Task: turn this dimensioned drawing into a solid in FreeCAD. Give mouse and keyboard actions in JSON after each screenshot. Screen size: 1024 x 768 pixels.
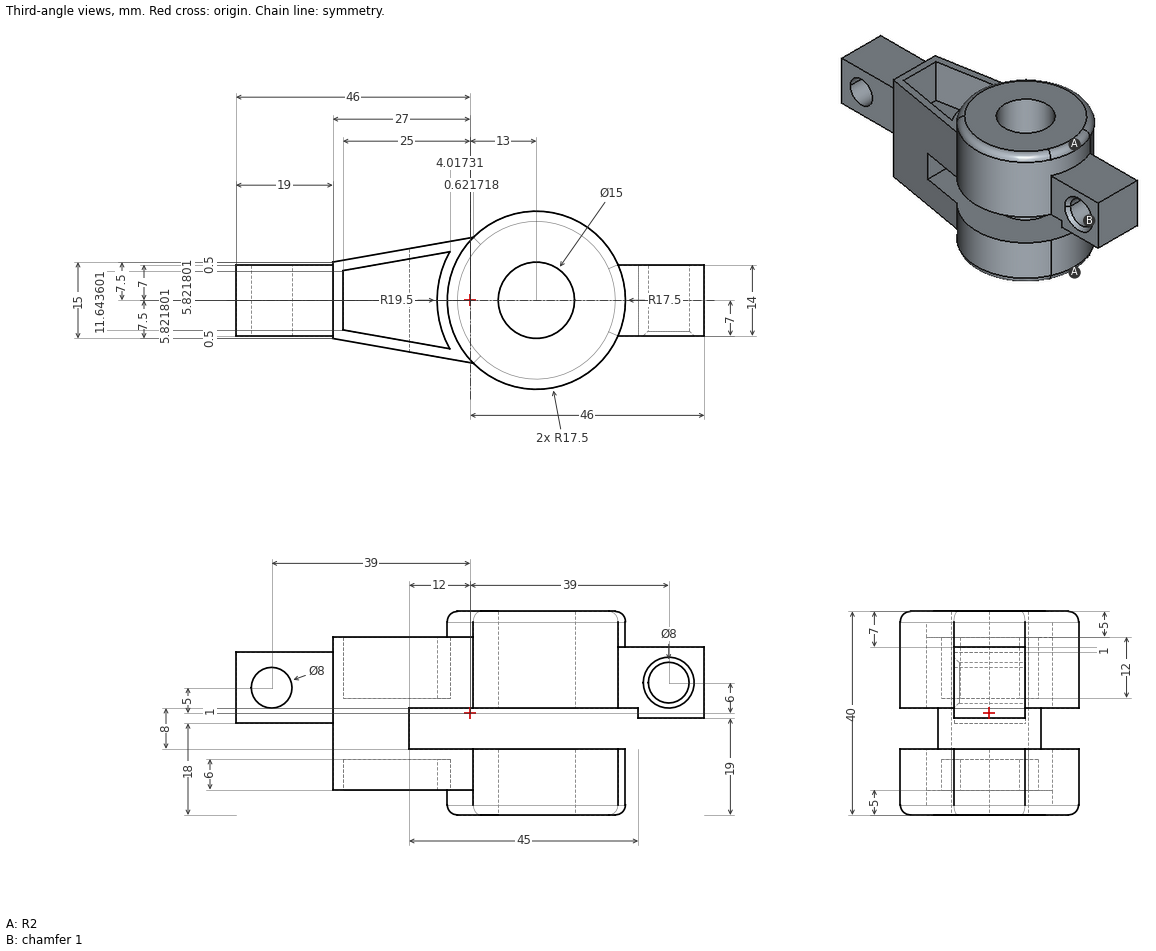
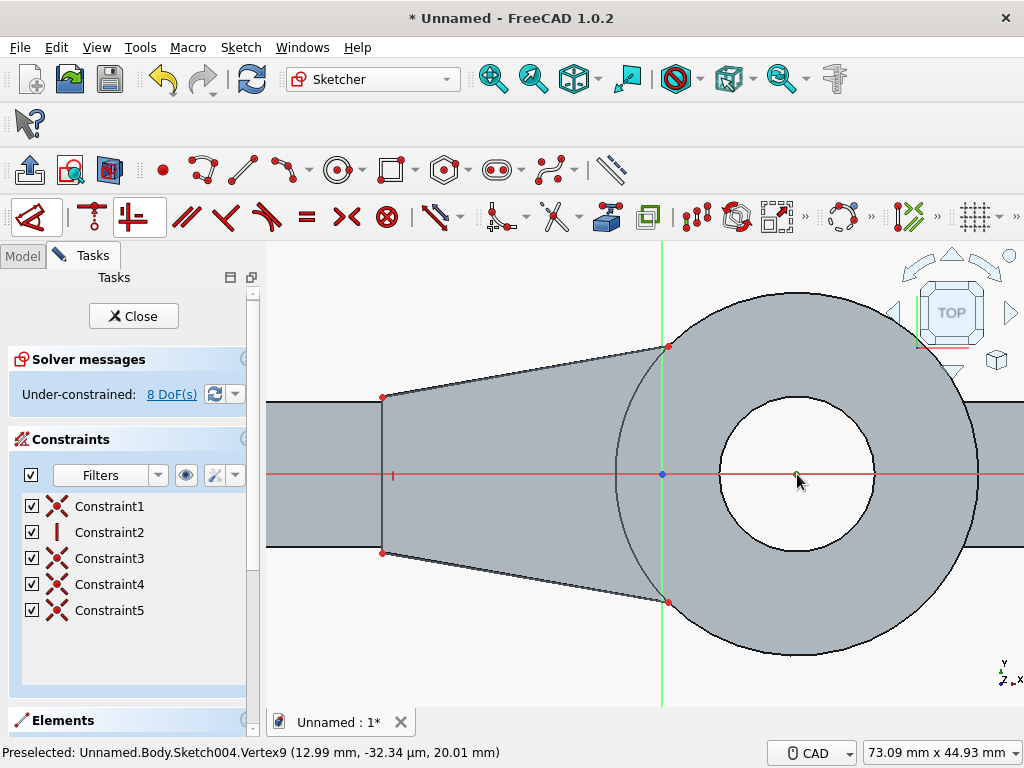
{"action": "left_click", "coordinate": [334, 474]}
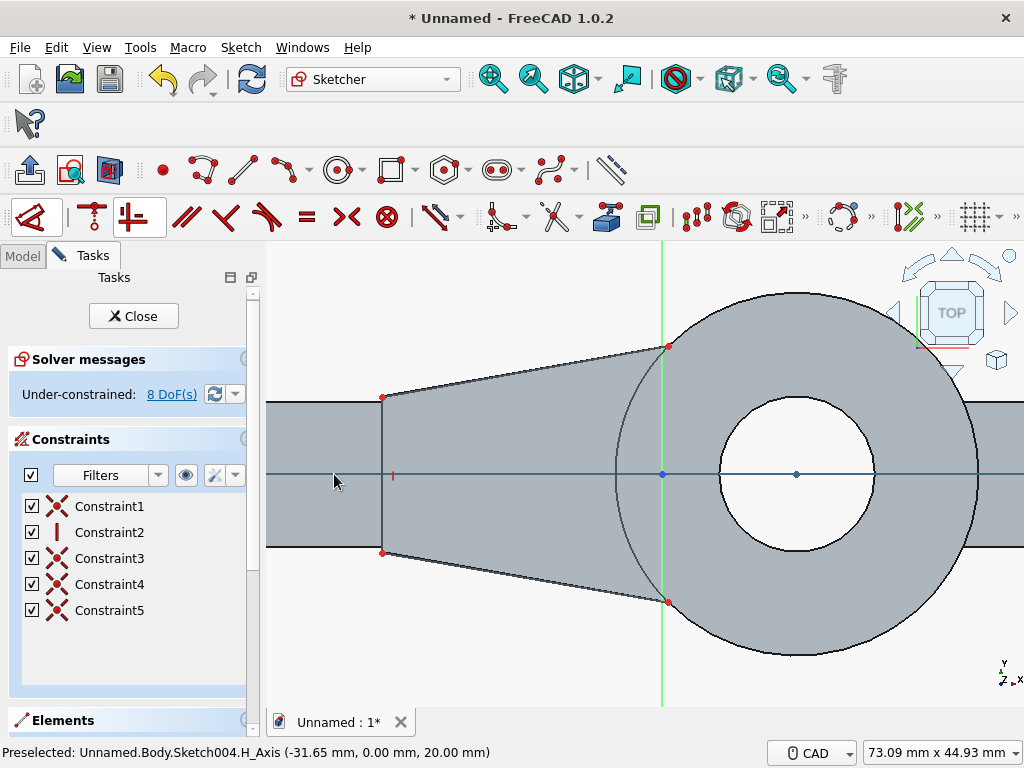
{"action": "left_click", "coordinate": [92, 218]}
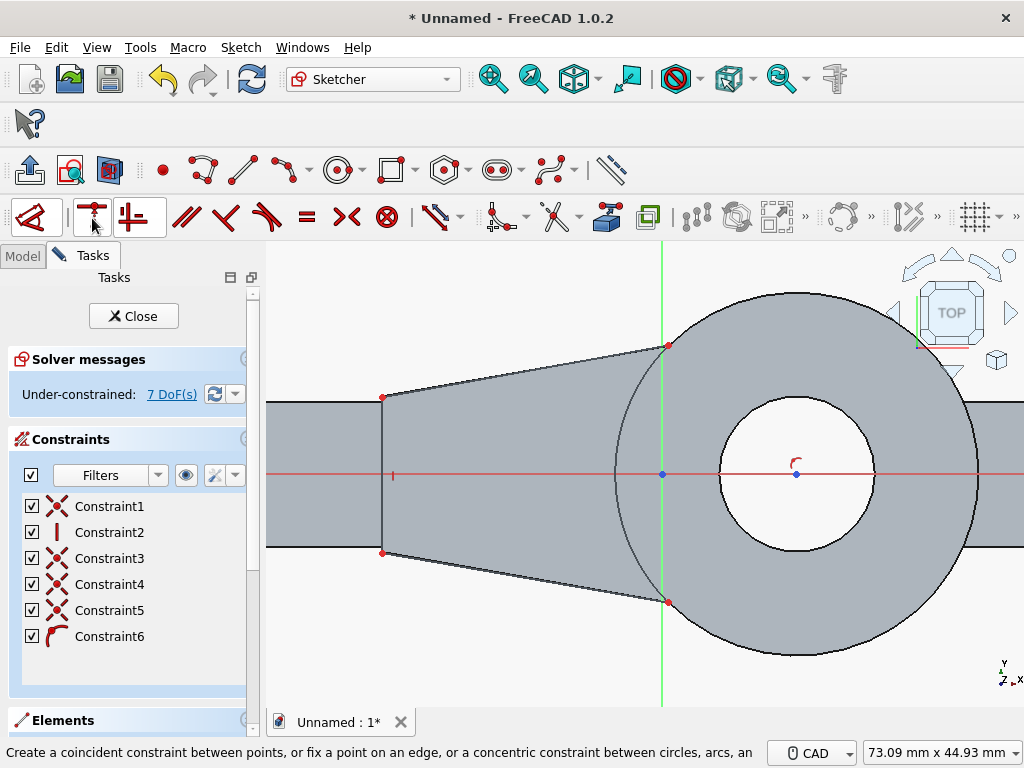
{"action": "left_click", "coordinate": [624, 418]}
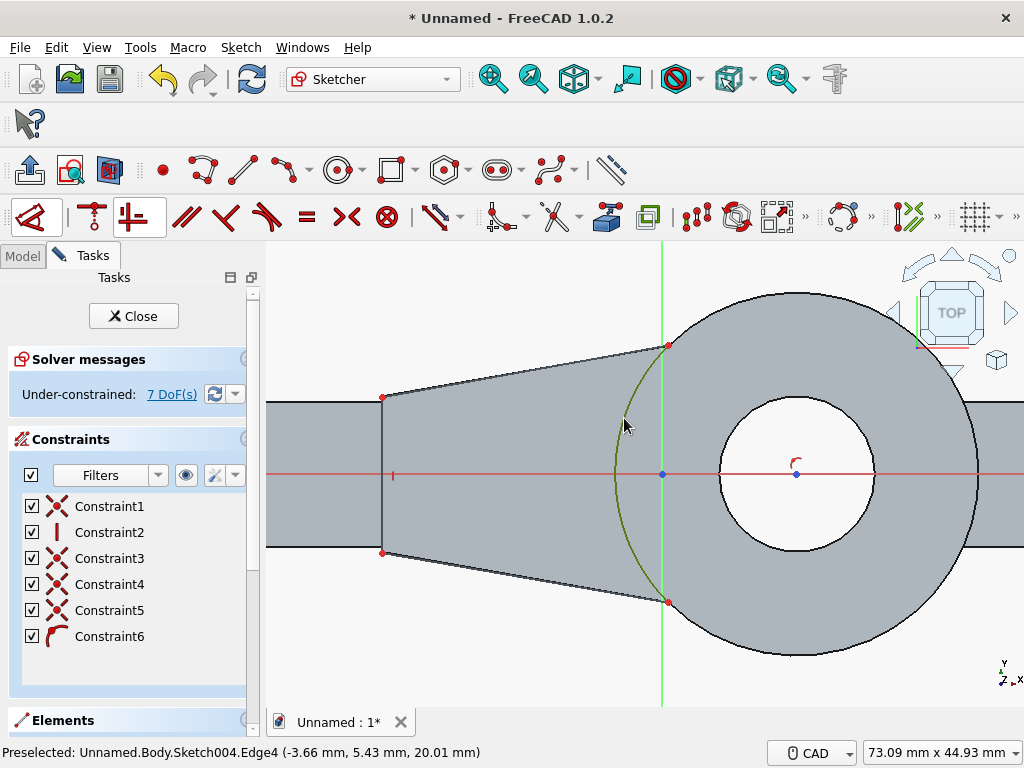
{"action": "key", "text": "k r"}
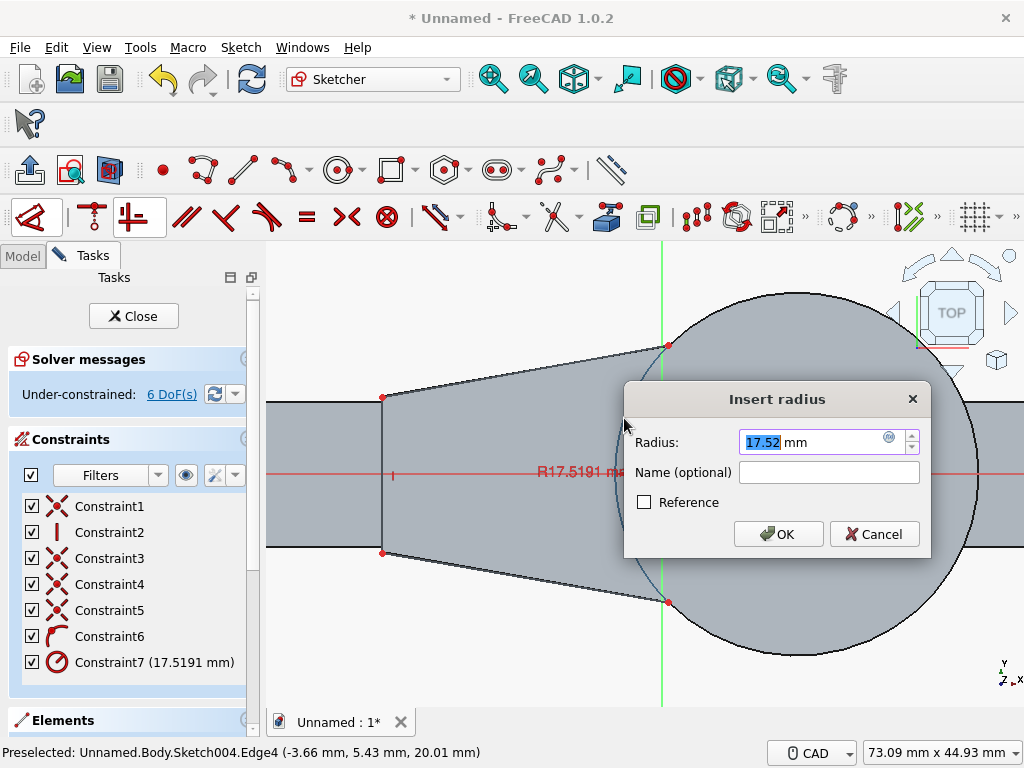
{"action": "type", "text": "17.5"}
{"action": "key", "text": "Return"}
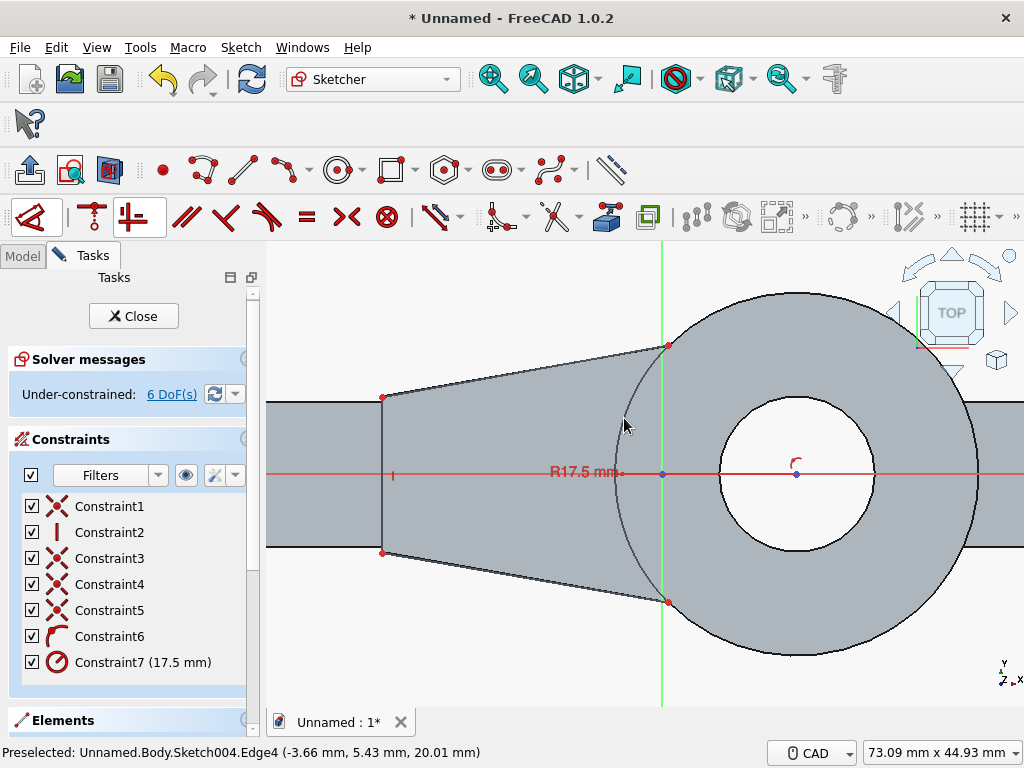
{"action": "left_click", "coordinate": [382, 444]}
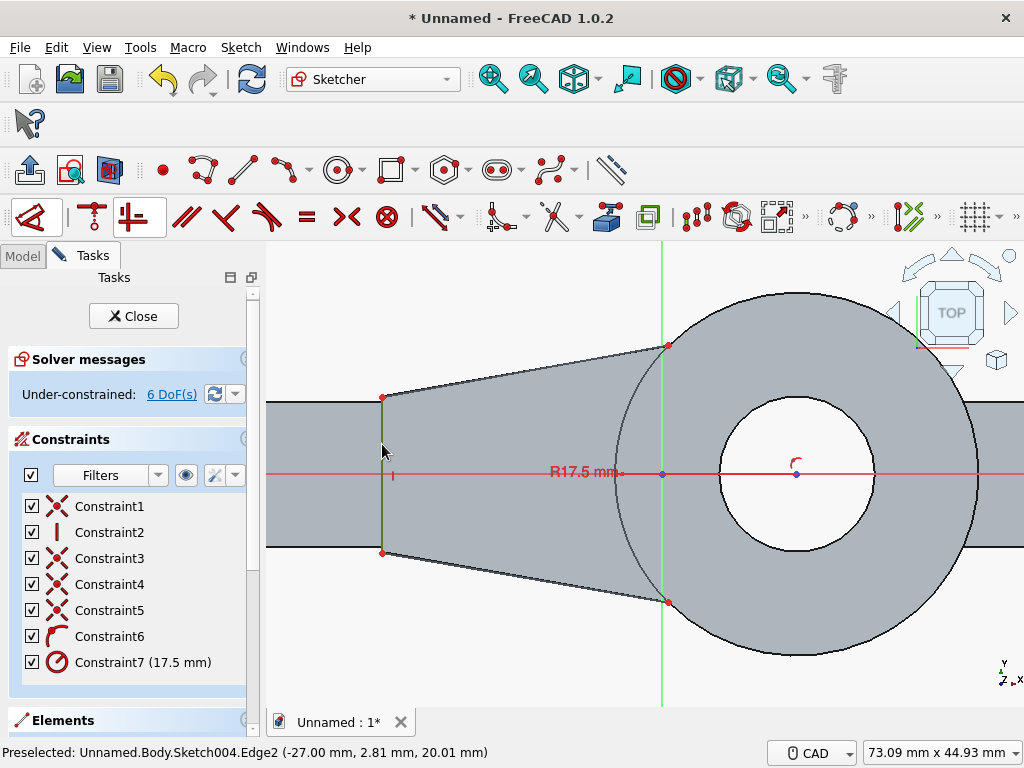
{"action": "left_click", "coordinate": [56, 218]}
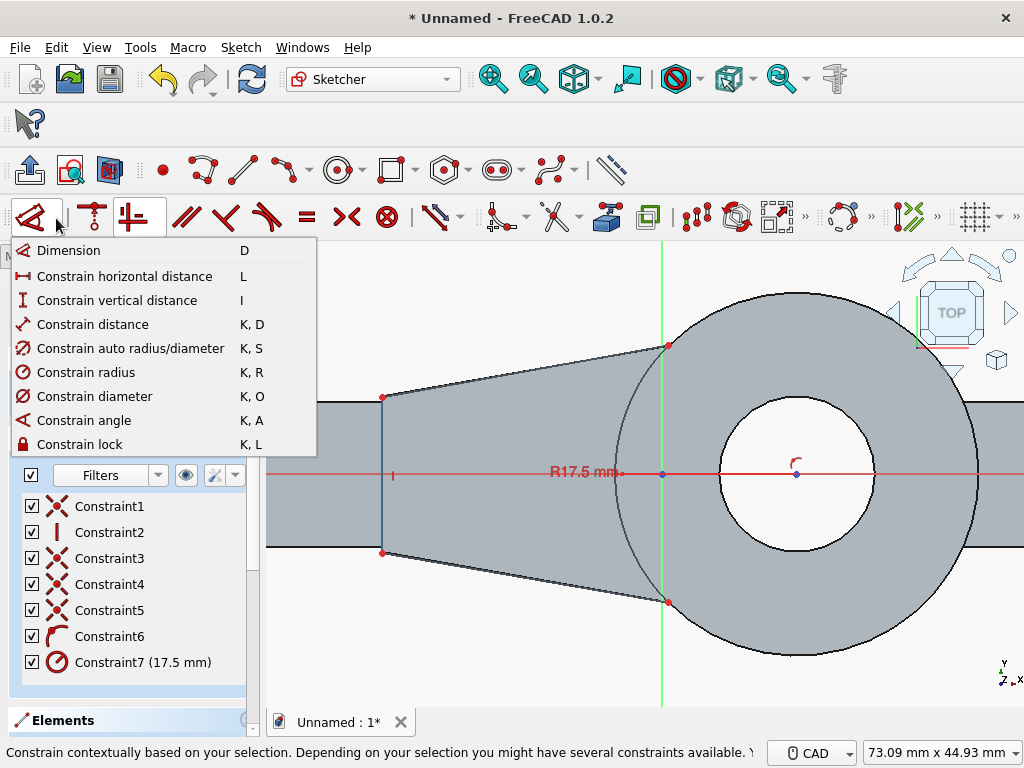
{"action": "left_click", "coordinate": [164, 300]}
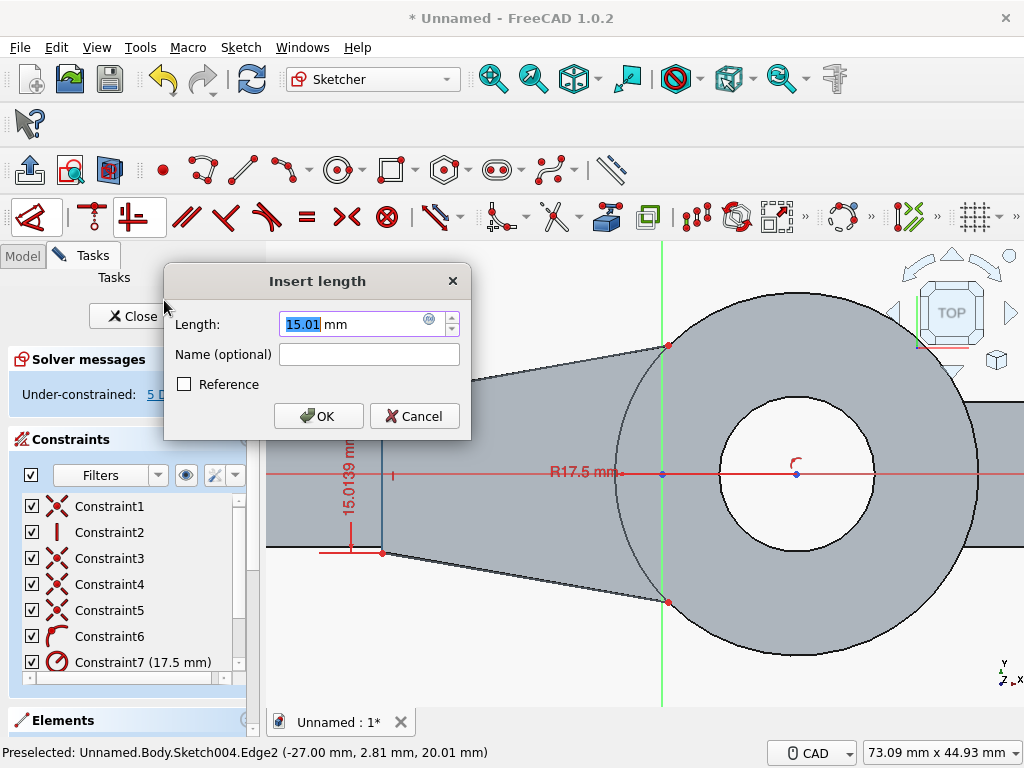
{"action": "type", "text": "15"}
{"action": "key", "text": "Return"}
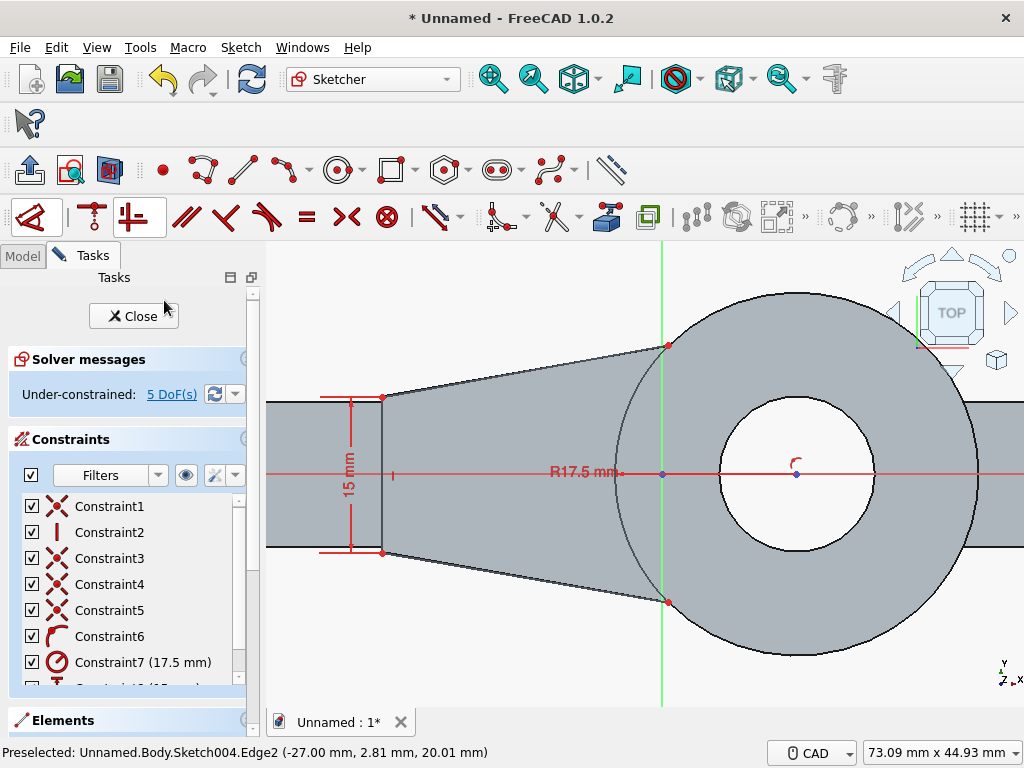
{"action": "left_click", "coordinate": [382, 397]}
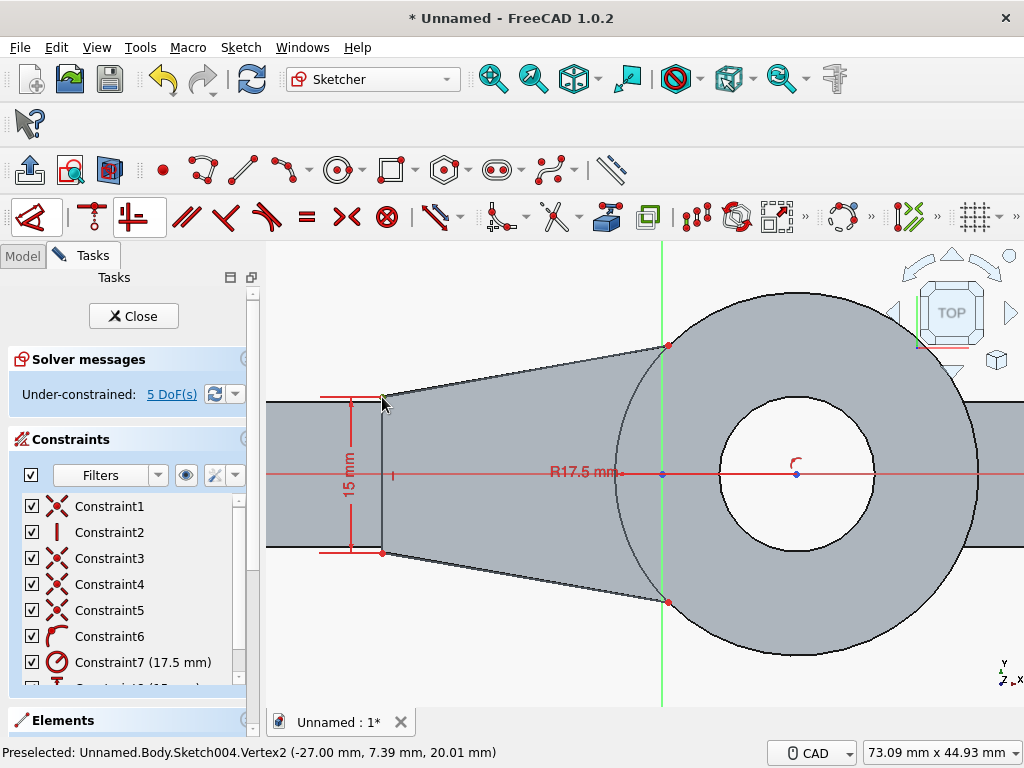
{"action": "left_click", "coordinate": [56, 218]}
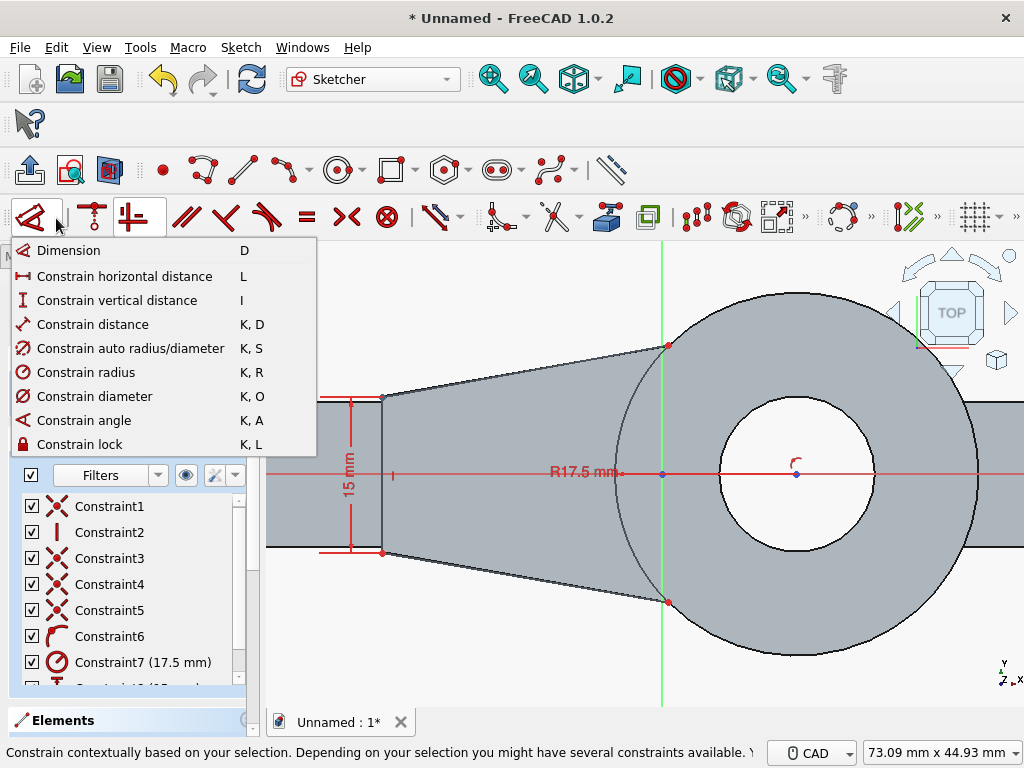
{"action": "left_click", "coordinate": [164, 276]}